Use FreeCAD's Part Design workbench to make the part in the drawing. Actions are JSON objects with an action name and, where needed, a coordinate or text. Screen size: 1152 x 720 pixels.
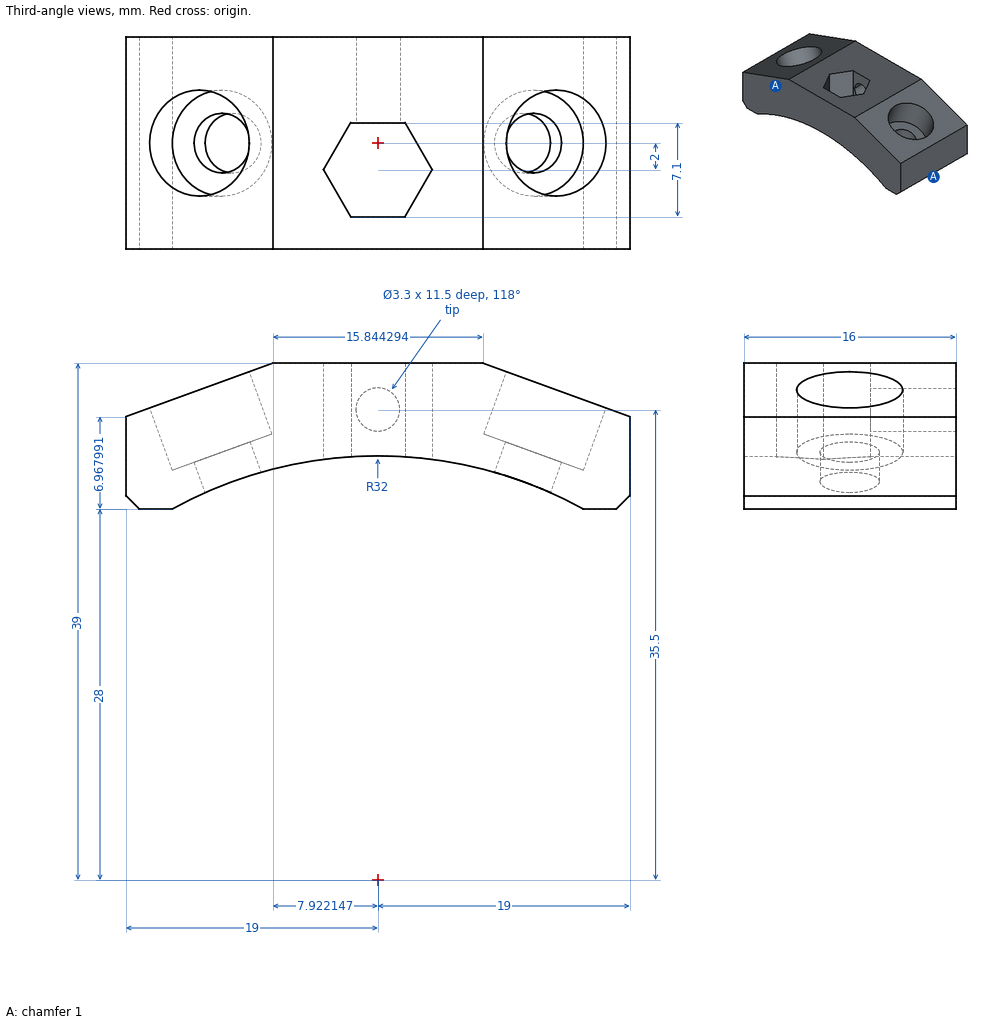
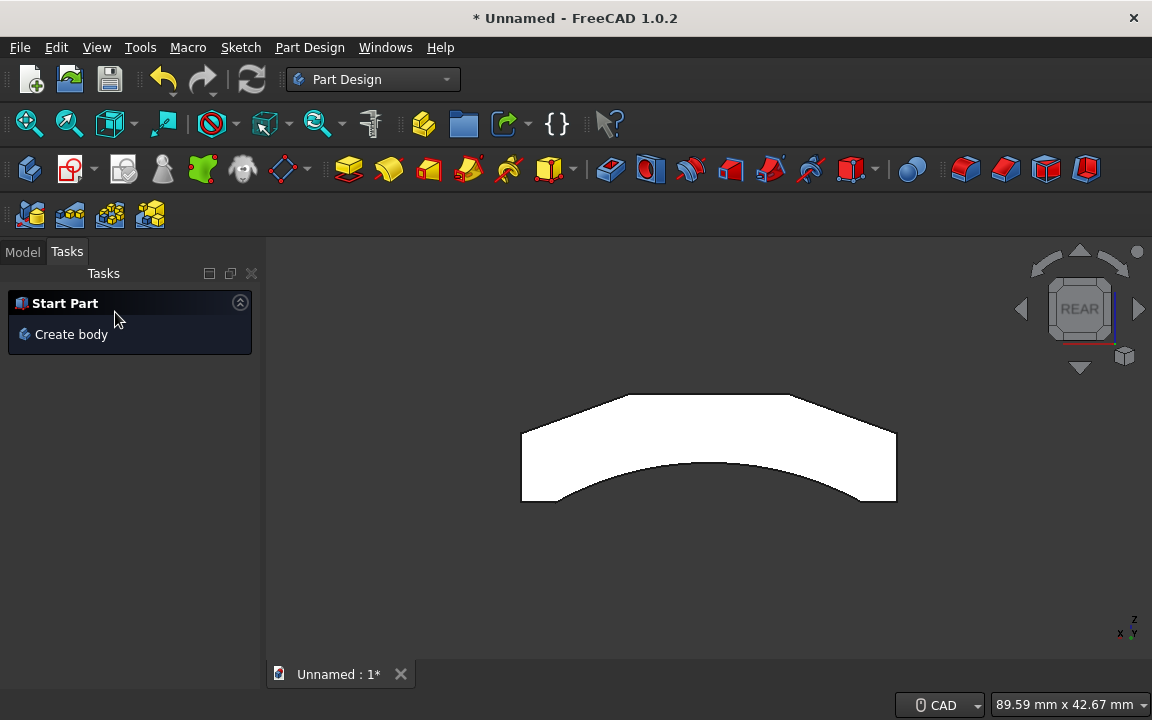
{"action": "left_click", "coordinate": [30, 124]}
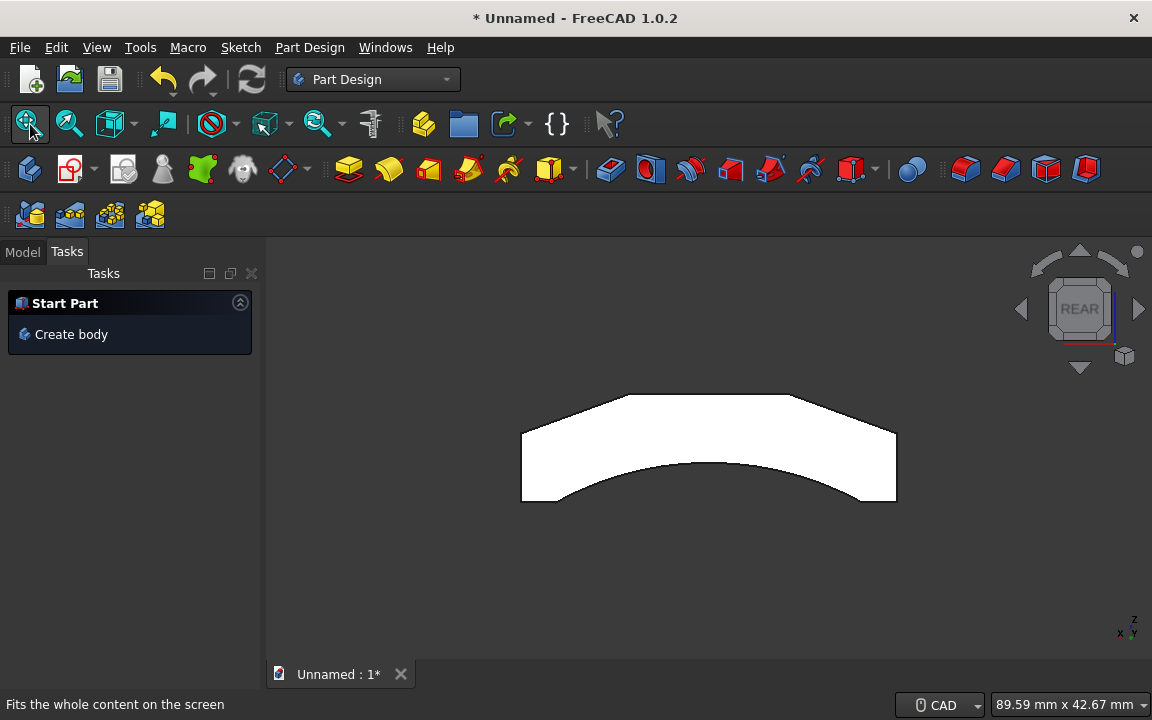
{"action": "left_click", "coordinate": [655, 431]}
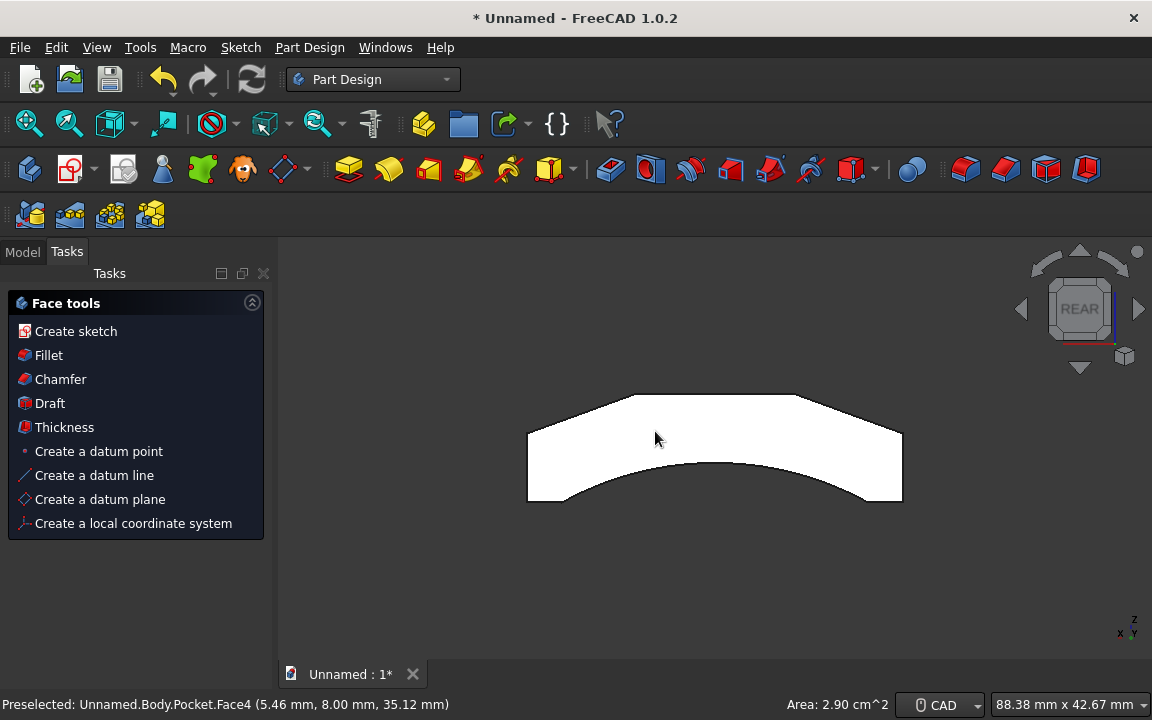
{"action": "left_click", "coordinate": [70, 170]}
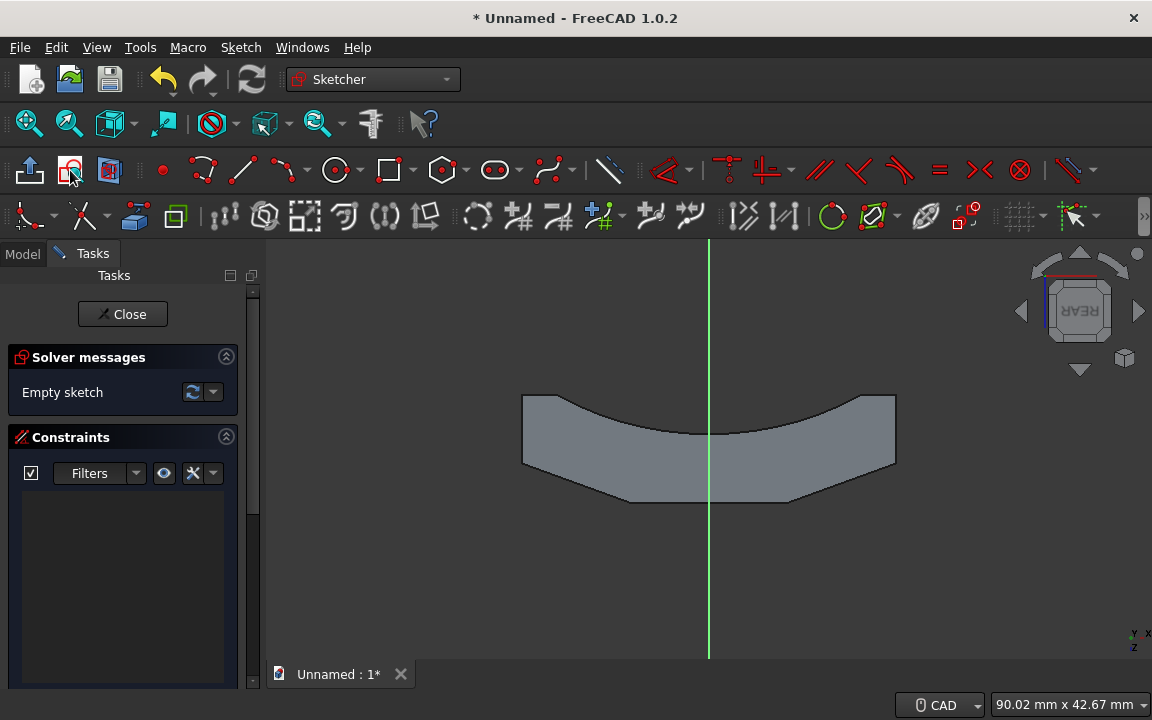
{"action": "scroll", "coordinate": [720, 472], "scroll_direction": "up", "scroll_amount": 10}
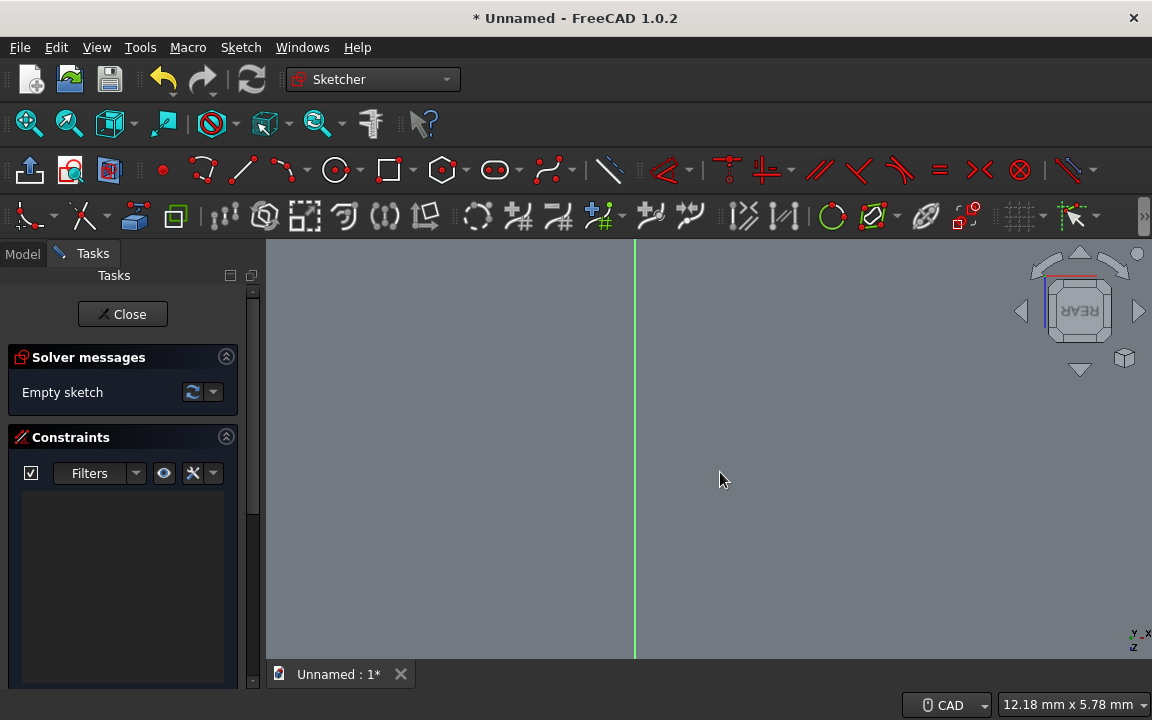
{"action": "key", "text": "g c"}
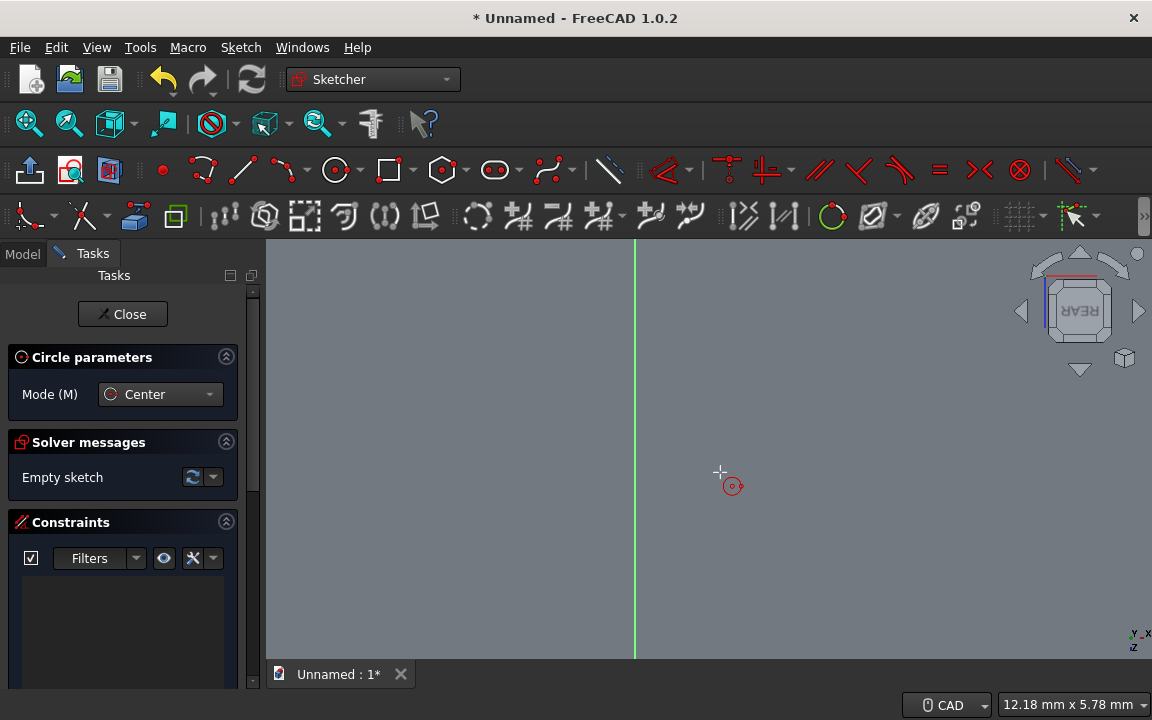
{"action": "left_click", "coordinate": [635, 444]}
{"action": "left_click", "coordinate": [720, 359]}
{"action": "key", "text": "Escape"}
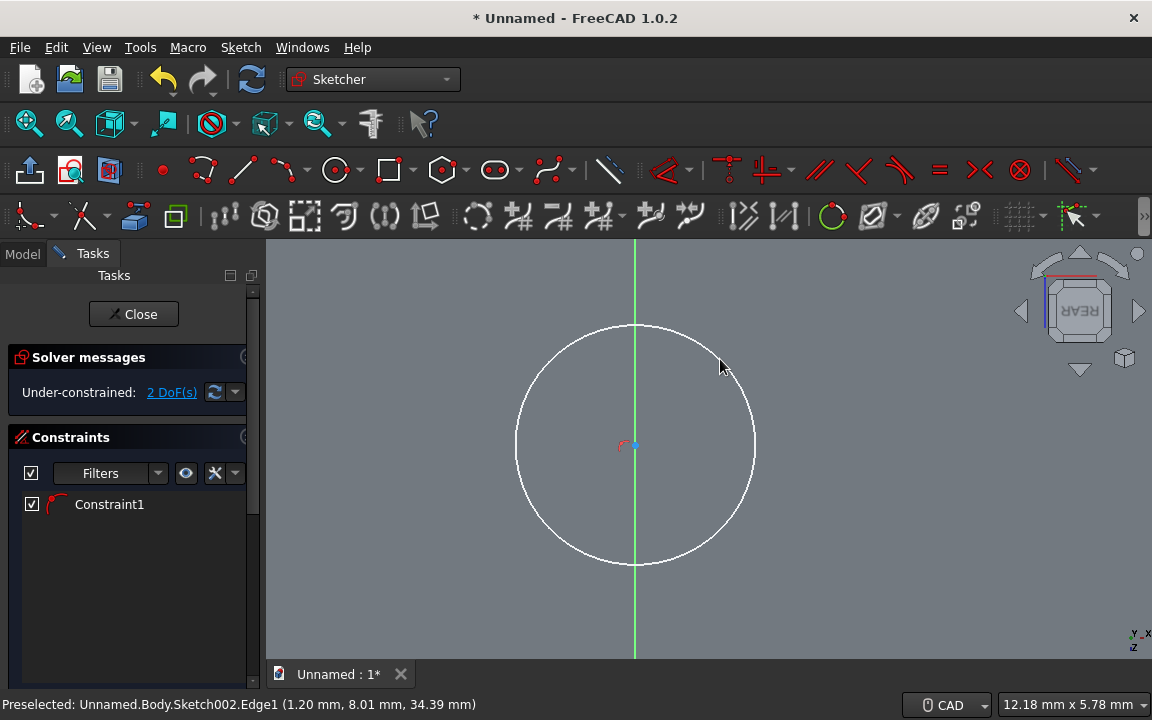
{"action": "key", "text": "d"}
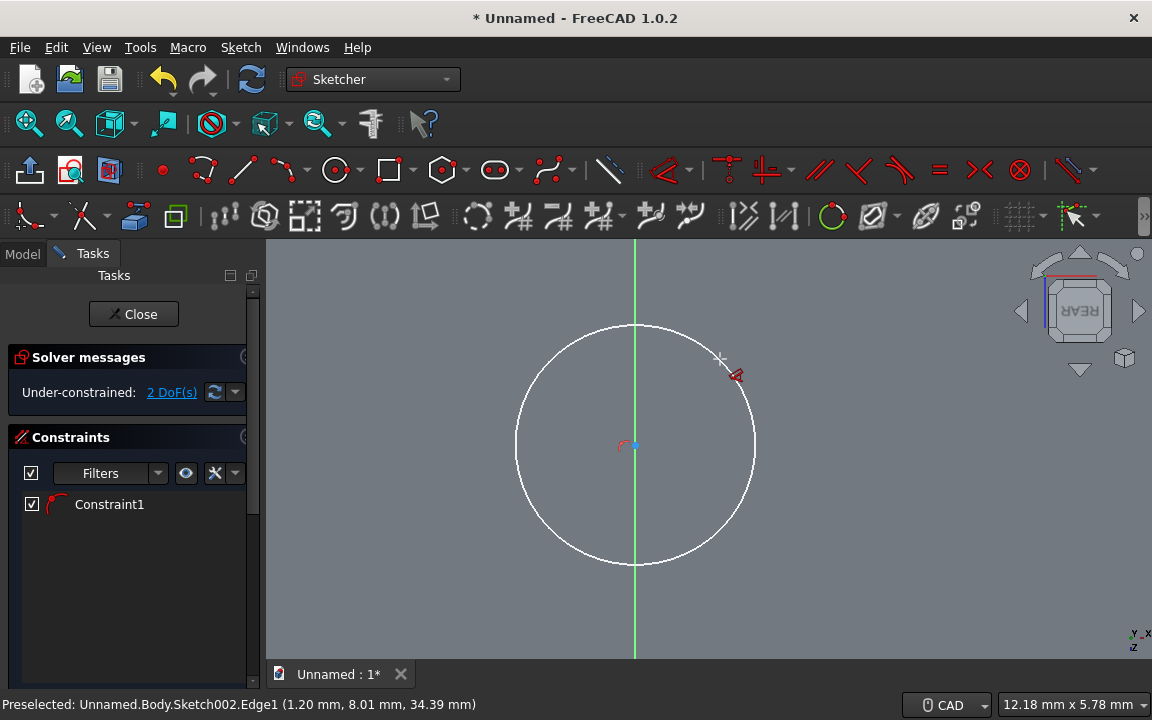
{"action": "left_click", "coordinate": [720, 360]}
{"action": "left_click", "coordinate": [743, 337]}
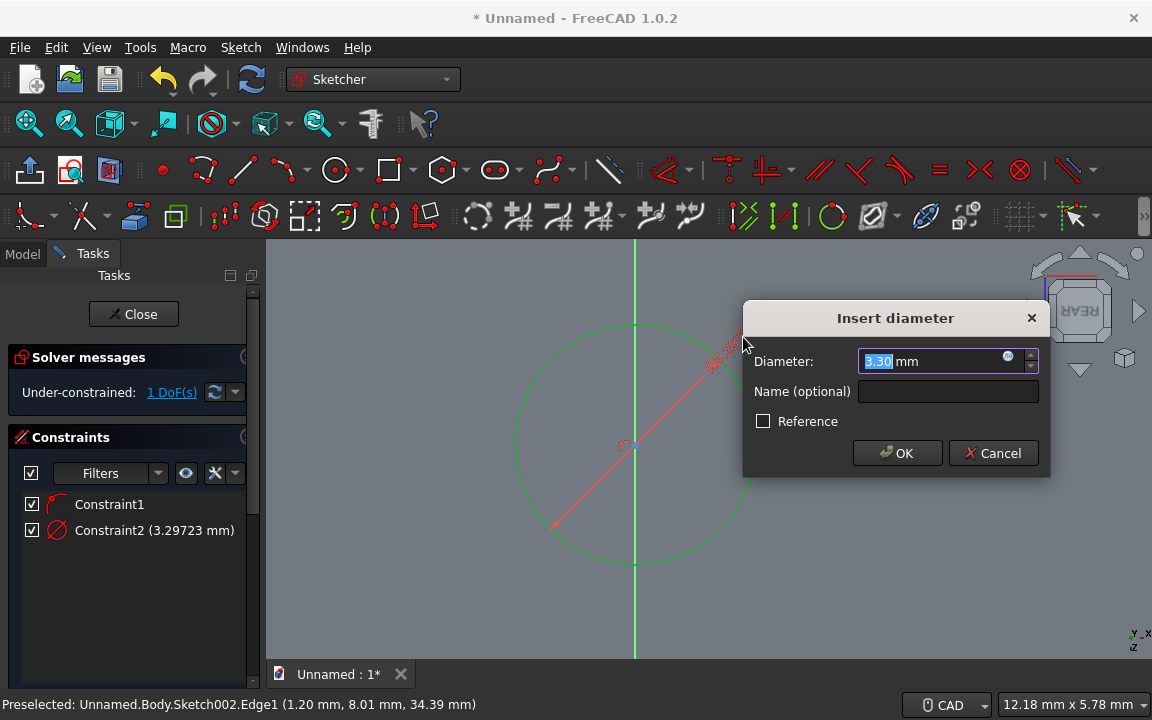
{"action": "type", "text": "3.3"}
{"action": "key", "text": "Return"}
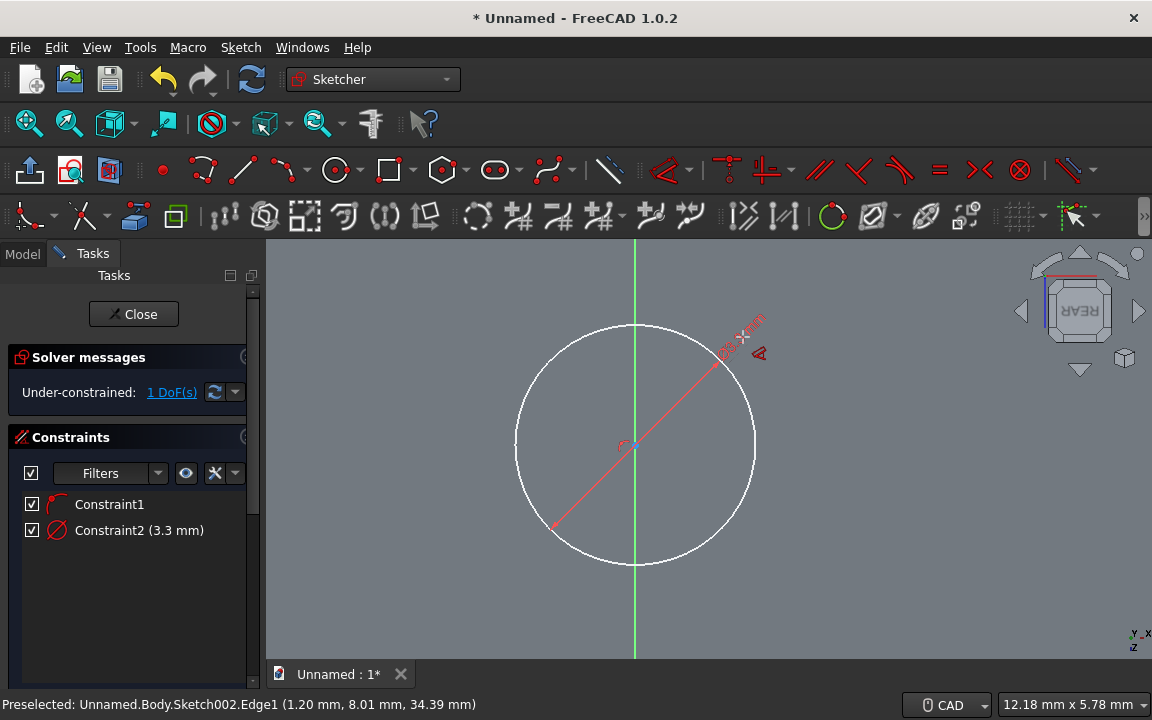
{"action": "left_click", "coordinate": [635, 445]}
{"action": "left_click", "coordinate": [669, 356]}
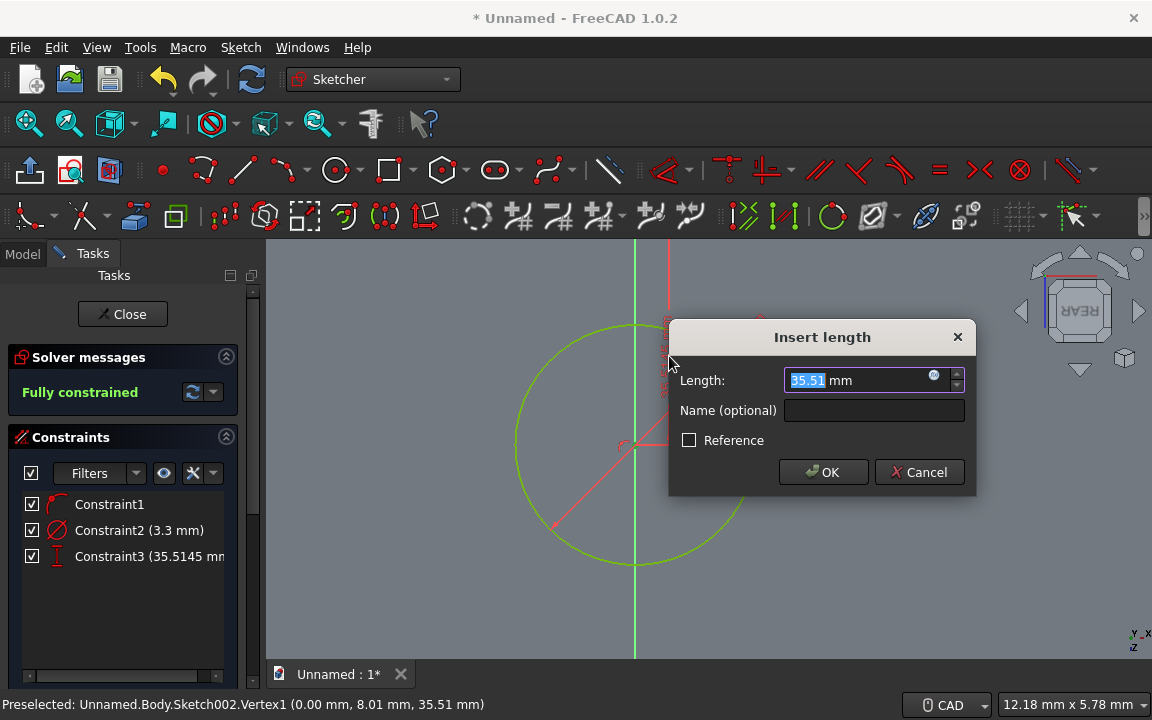
{"action": "type", "text": "35.5"}
{"action": "key", "text": "Return"}
{"action": "key", "text": "Escape"}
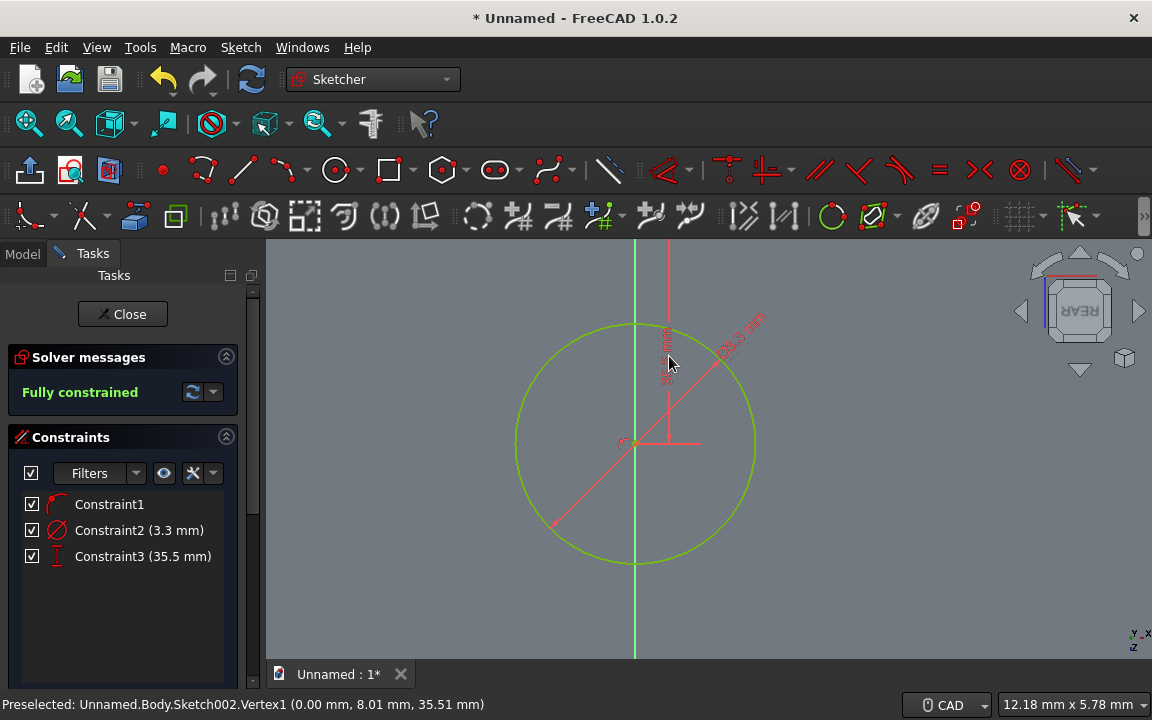
{"action": "left_click", "coordinate": [123, 314]}